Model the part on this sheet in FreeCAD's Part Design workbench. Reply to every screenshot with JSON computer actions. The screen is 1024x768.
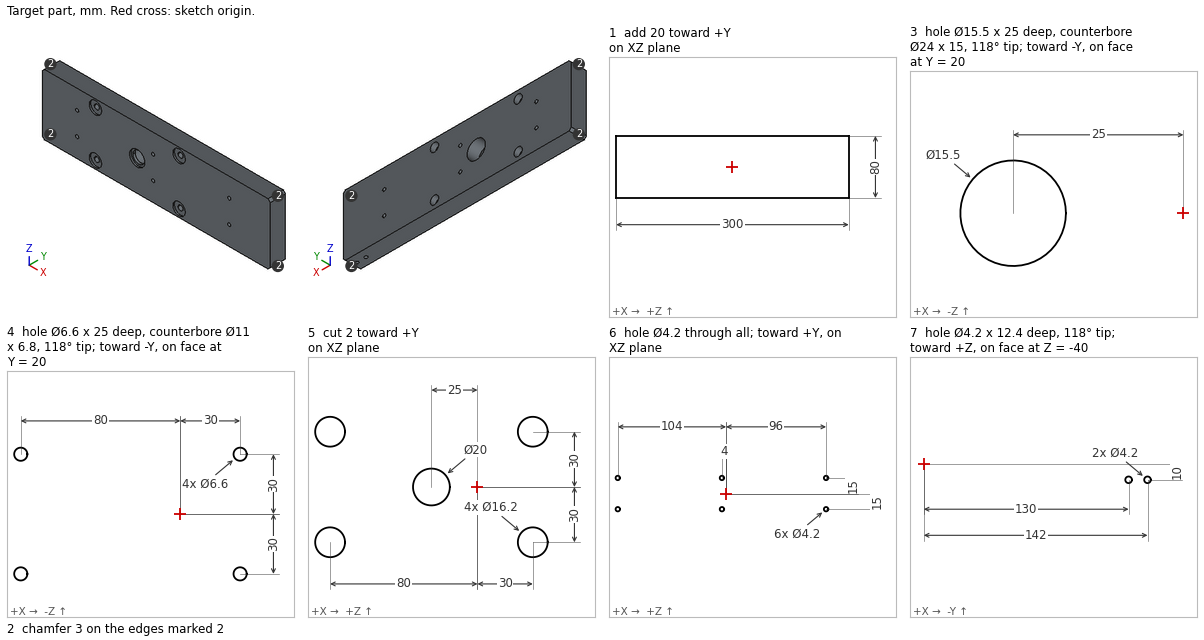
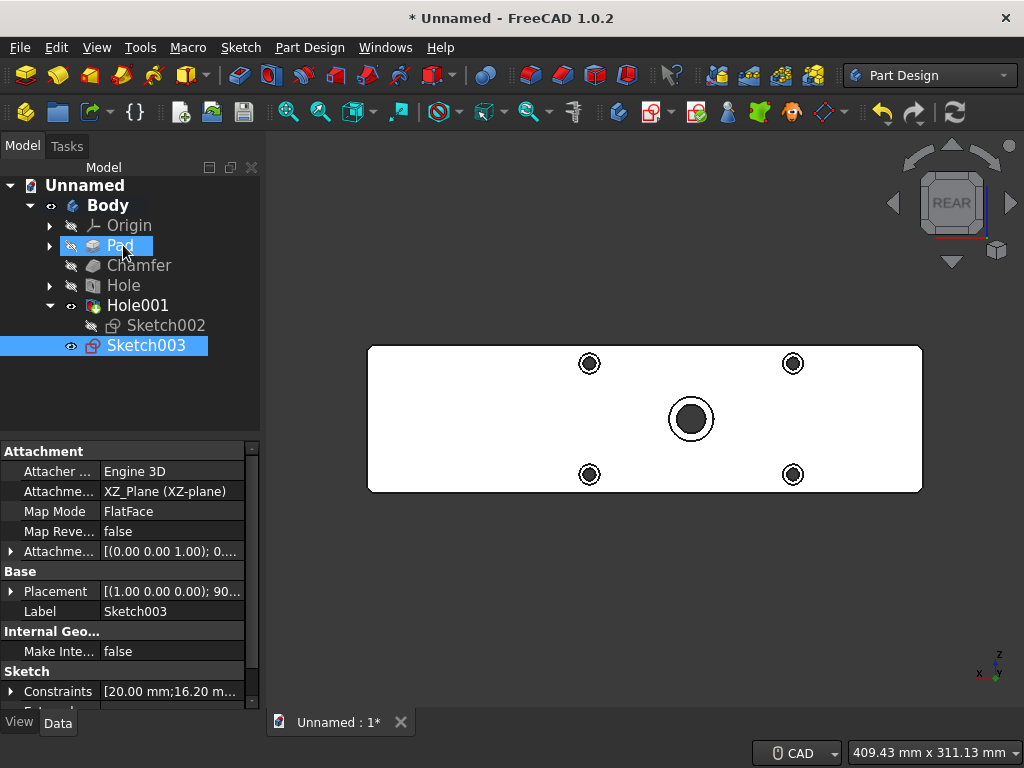
{"action": "left_click", "coordinate": [240, 76]}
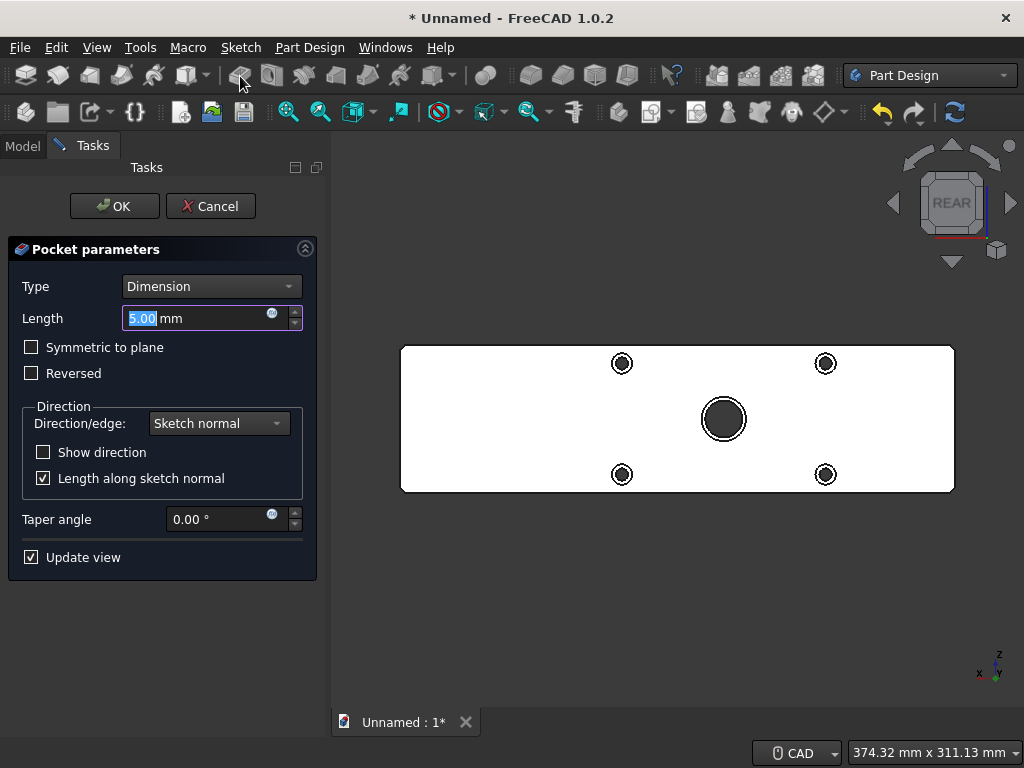
{"action": "type", "text": "2"}
{"action": "key", "text": "Tab"}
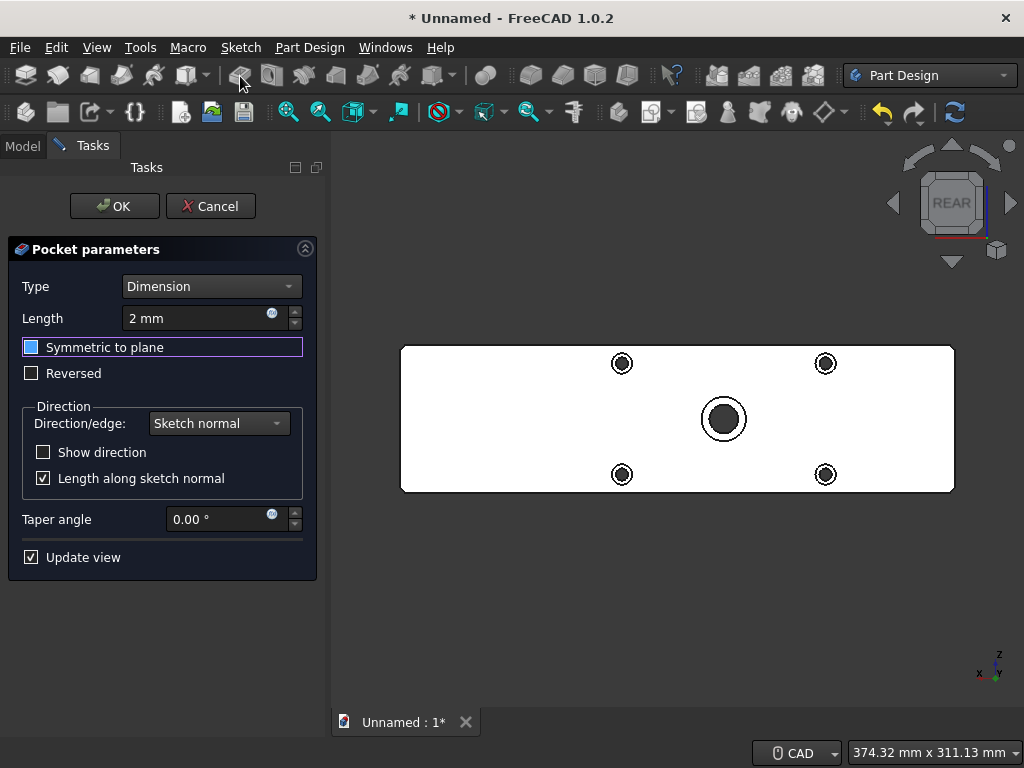
{"action": "left_click", "coordinate": [115, 206]}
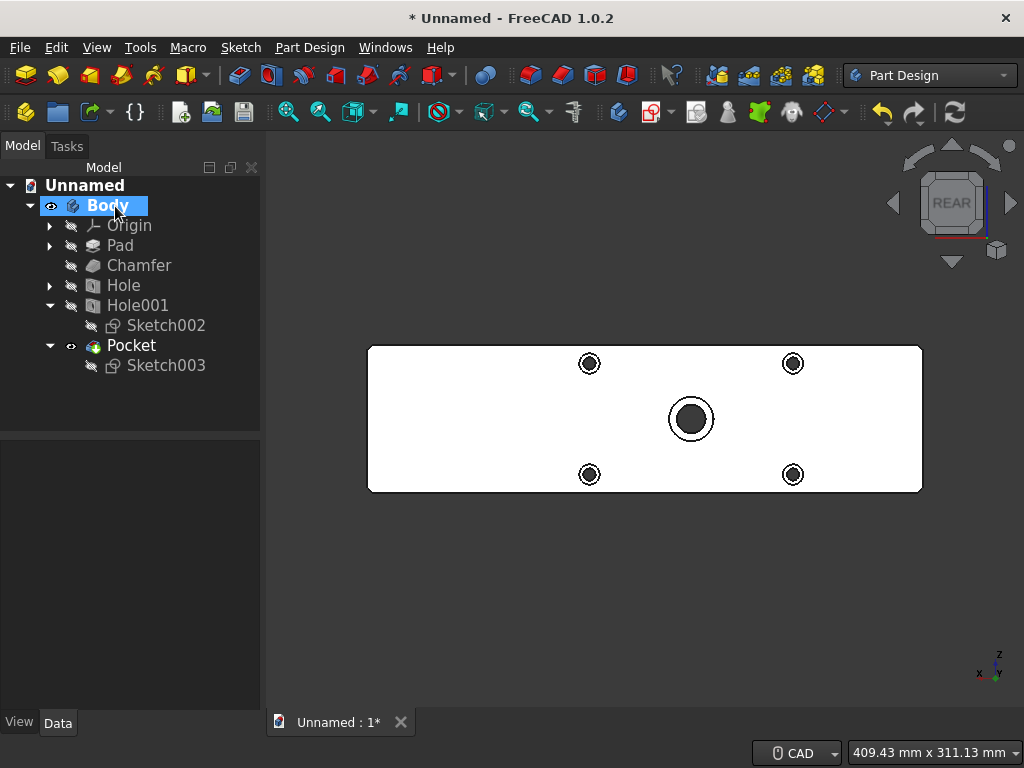
{"action": "left_click", "coordinate": [652, 112]}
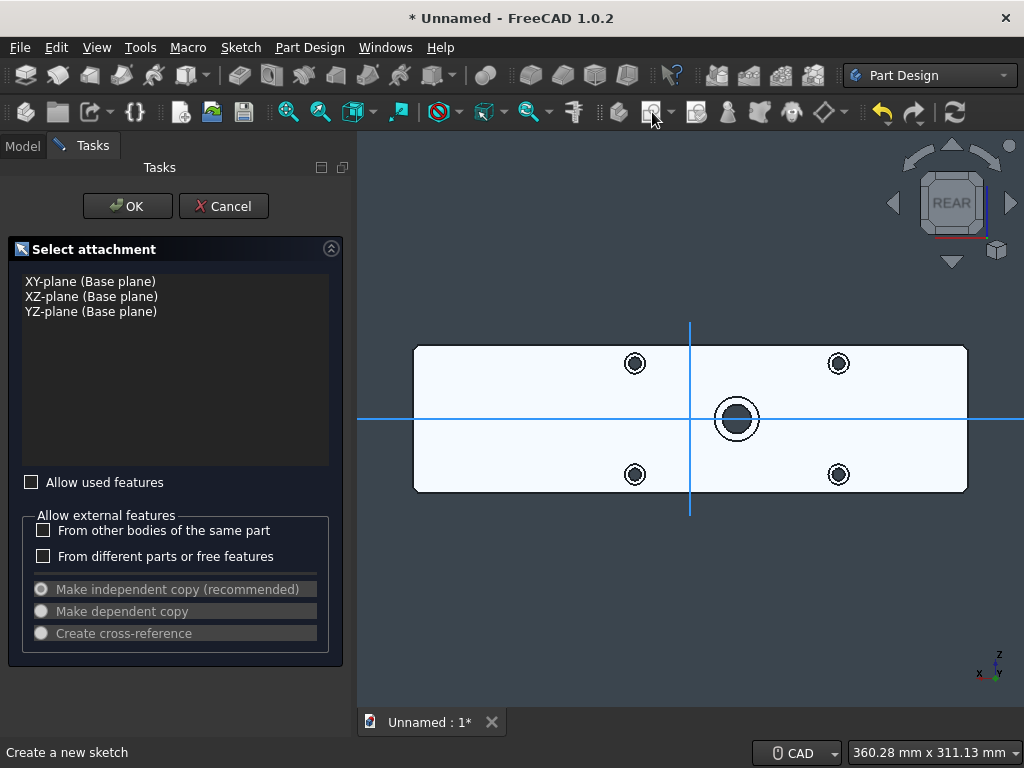
{"action": "left_click", "coordinate": [82, 296]}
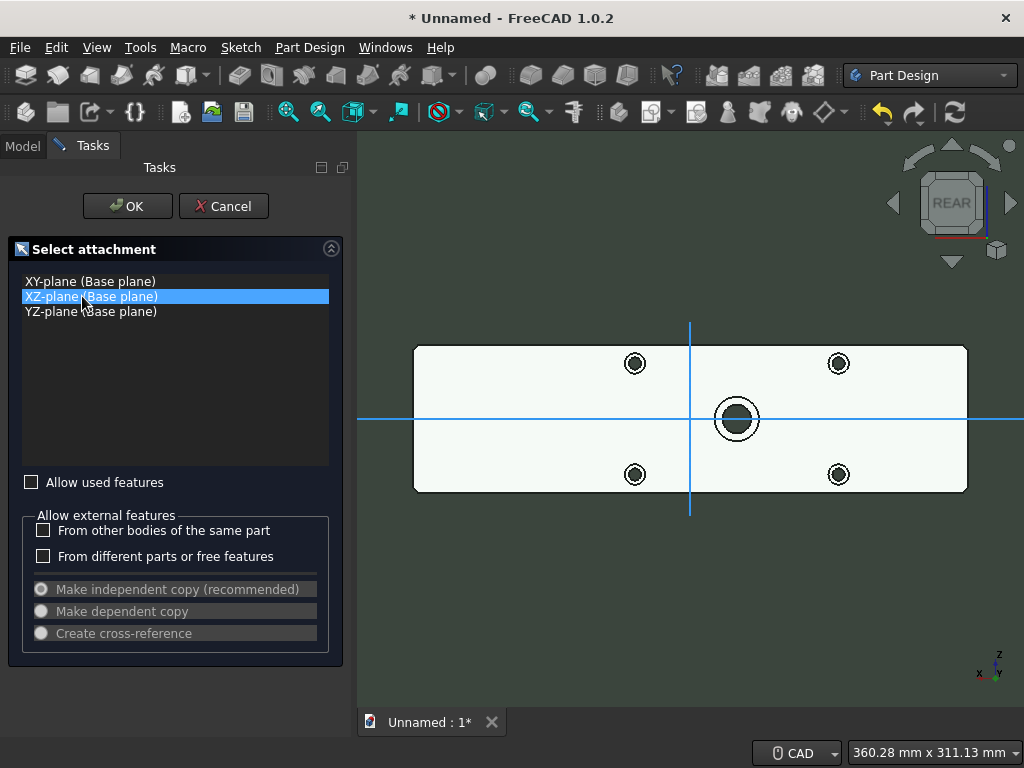
{"action": "left_click", "coordinate": [128, 206]}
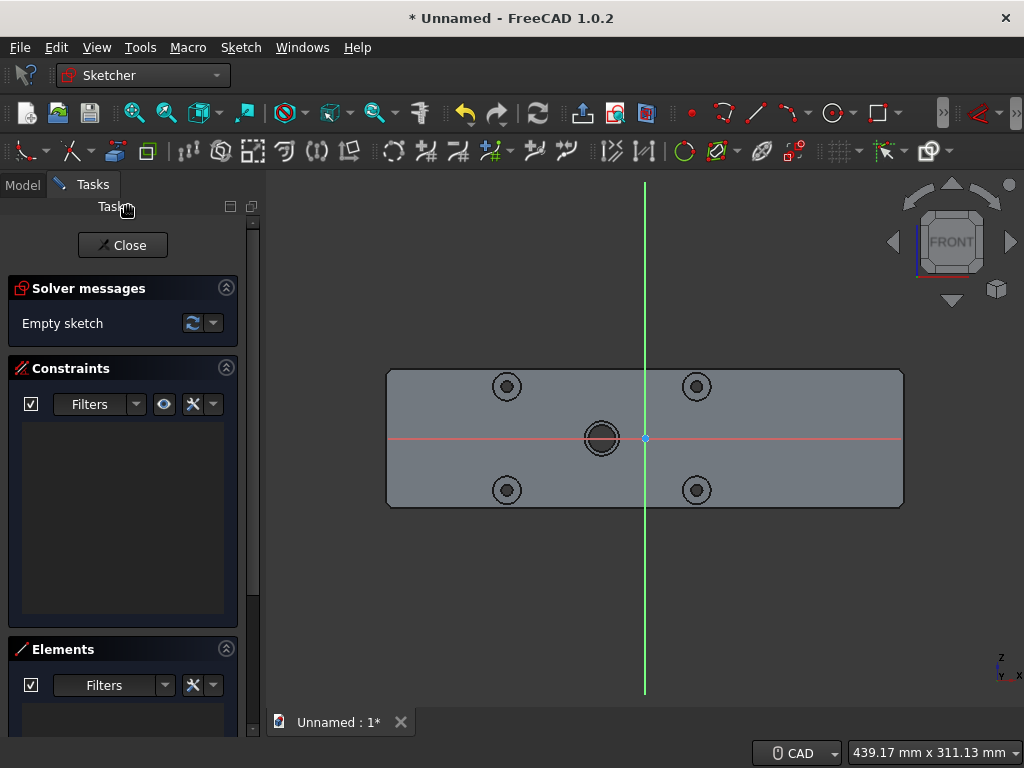
{"action": "left_click", "coordinate": [834, 114]}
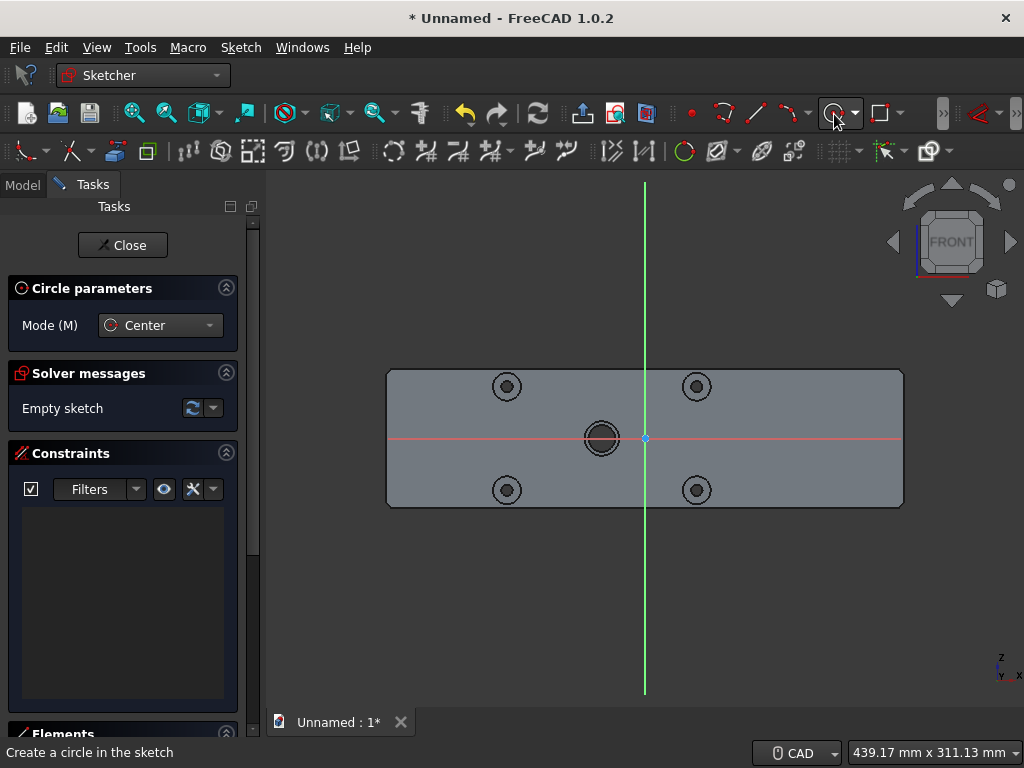
{"action": "scroll", "coordinate": [811, 413], "scroll_direction": "up", "scroll_amount": 10}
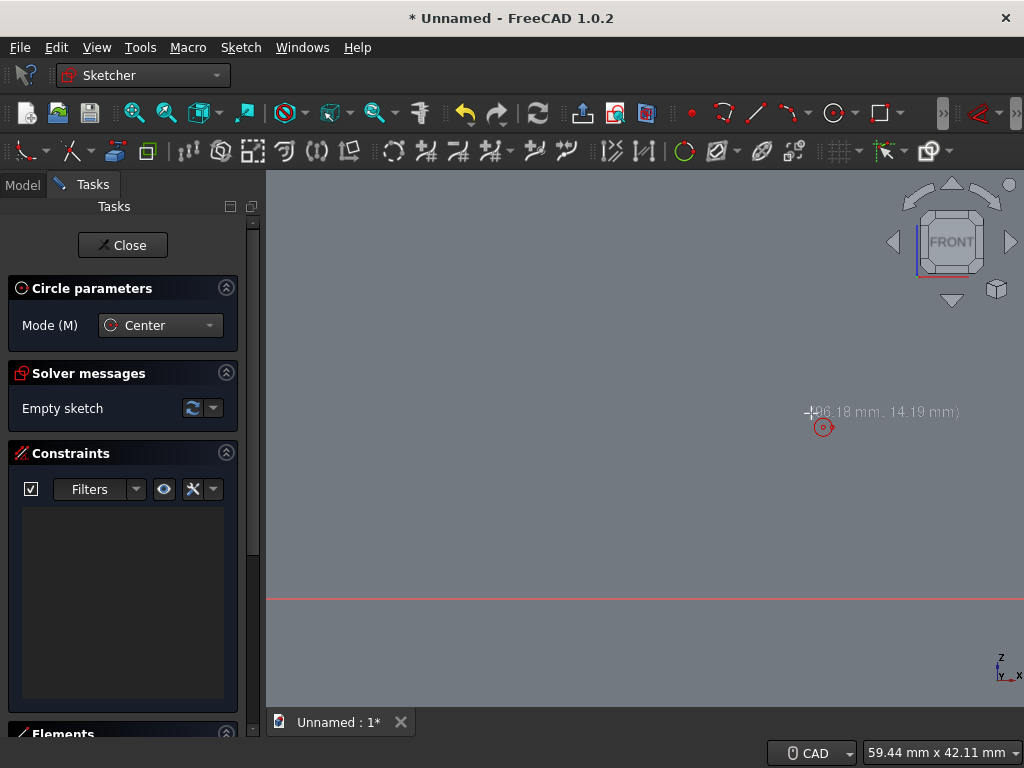
{"action": "scroll", "coordinate": [784, 407], "scroll_direction": "down", "scroll_amount": 9}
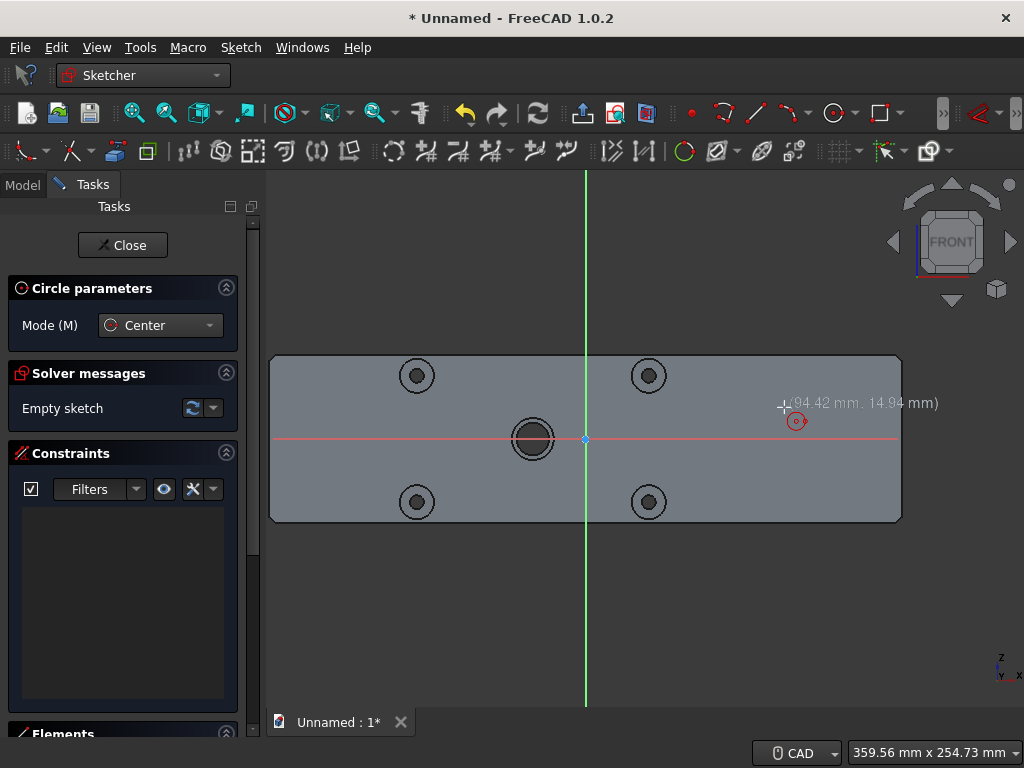
{"action": "left_click", "coordinate": [788, 407]}
{"action": "mouse_move", "coordinate": [791, 404]}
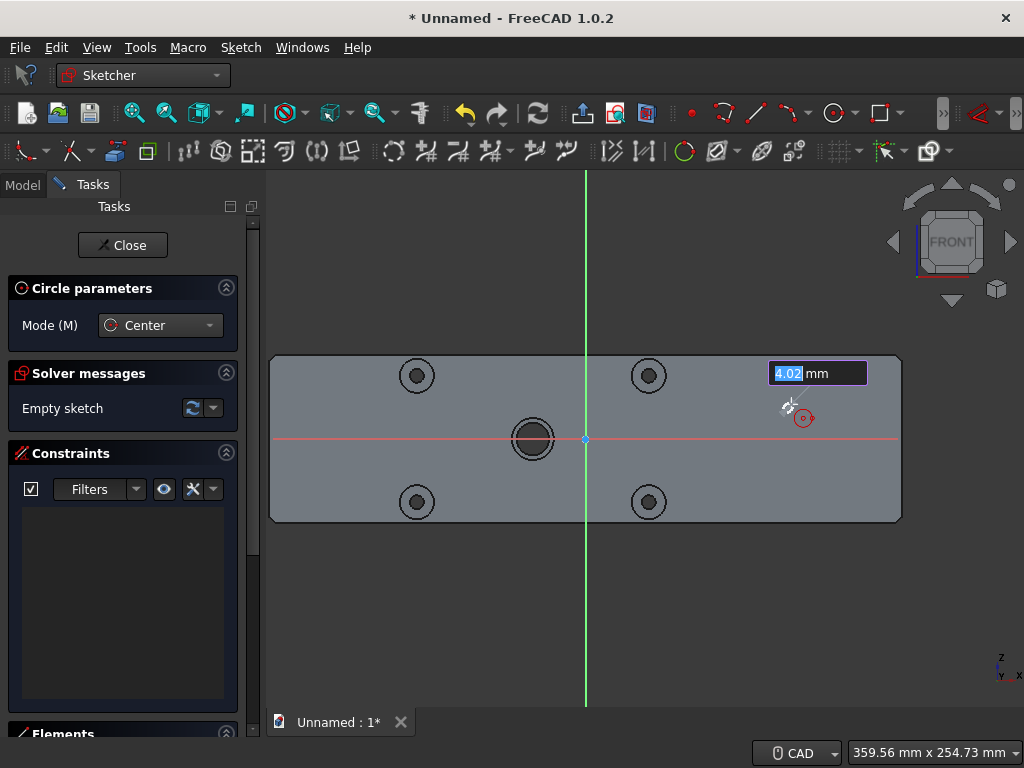
{"action": "type", "text": "4.2"}
{"action": "key", "text": "Return"}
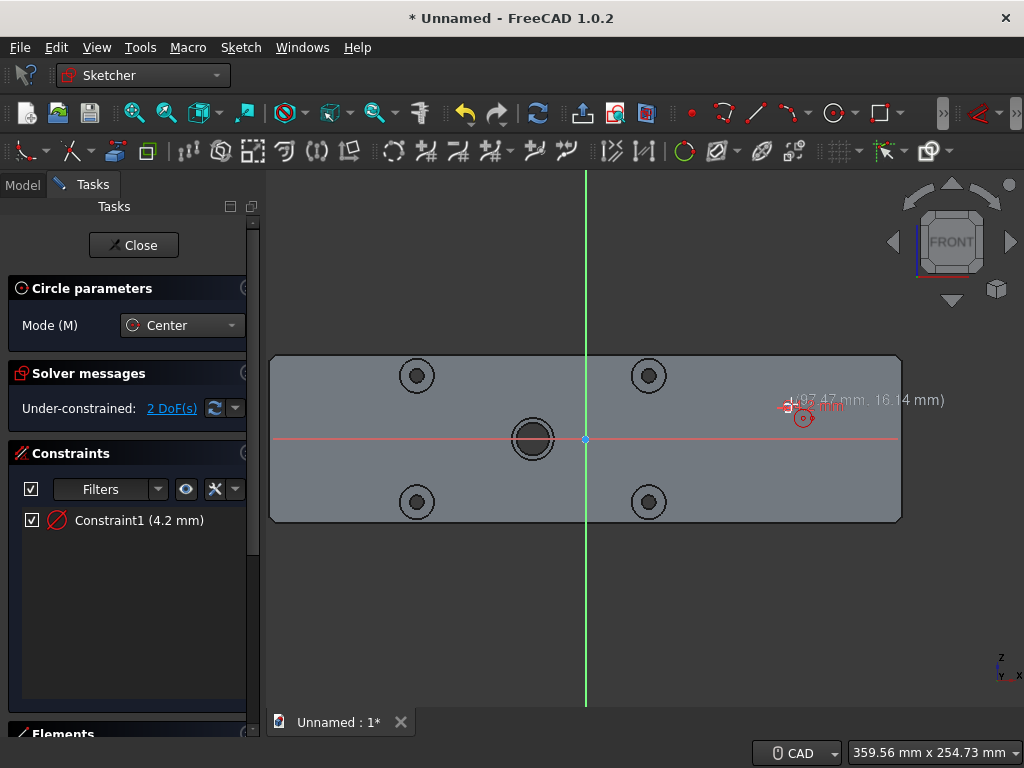
{"action": "scroll", "coordinate": [788, 471], "scroll_direction": "up", "scroll_amount": 9}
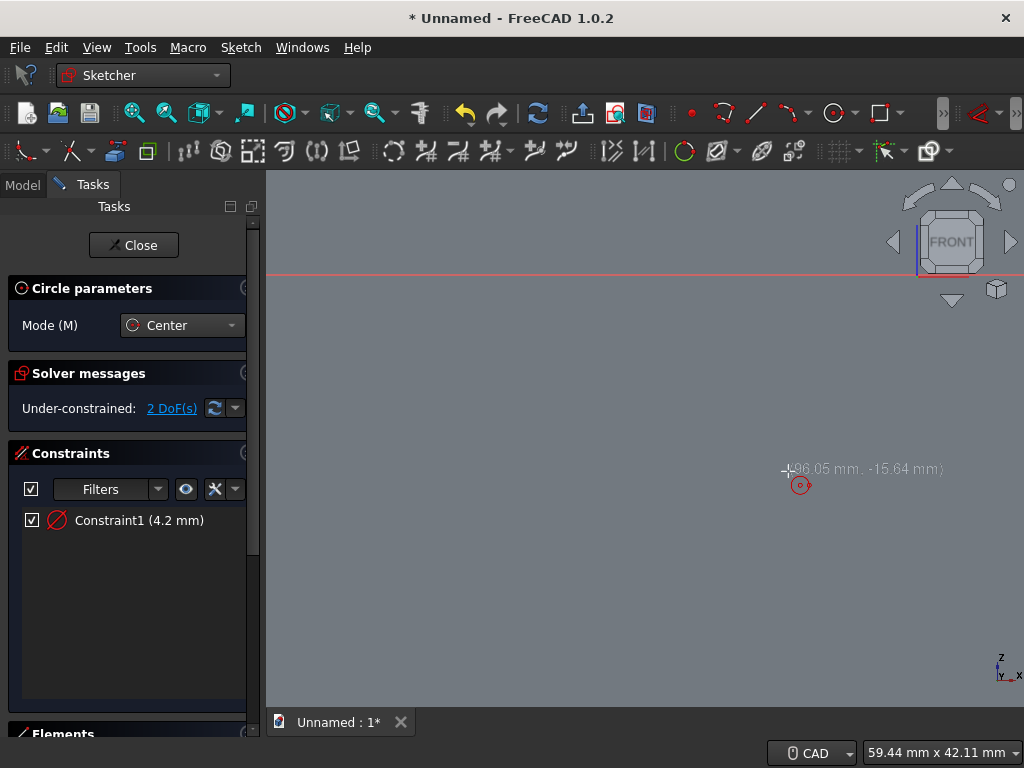
{"action": "scroll", "coordinate": [788, 471], "scroll_direction": "down", "scroll_amount": 9}